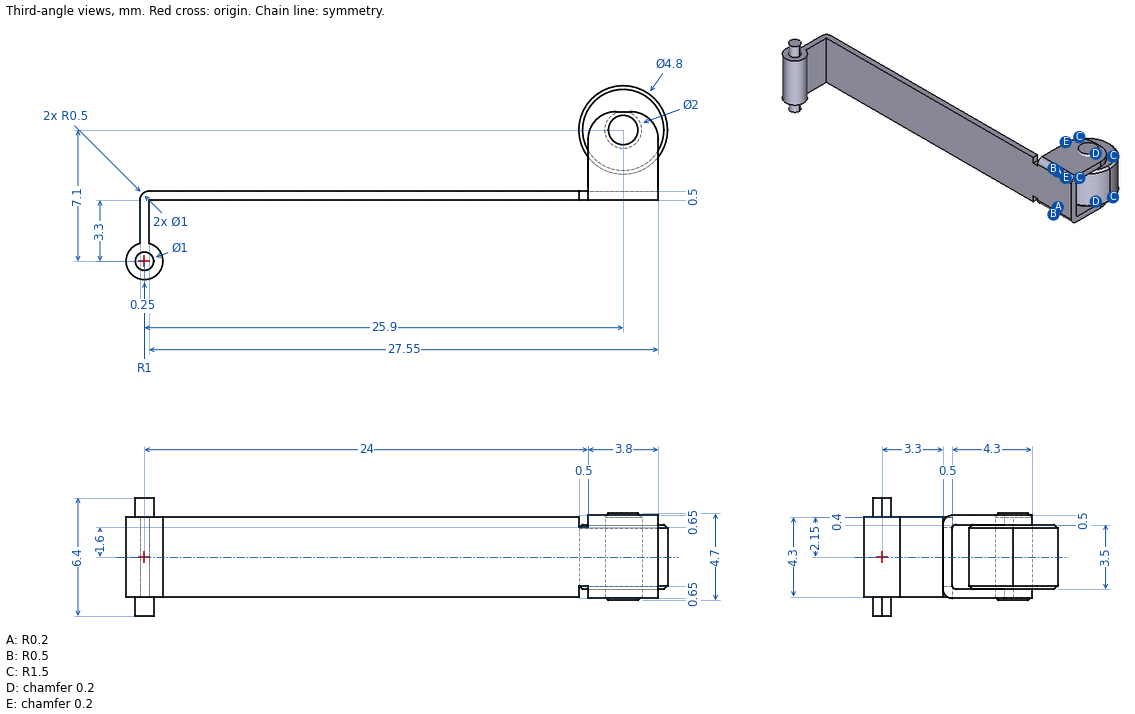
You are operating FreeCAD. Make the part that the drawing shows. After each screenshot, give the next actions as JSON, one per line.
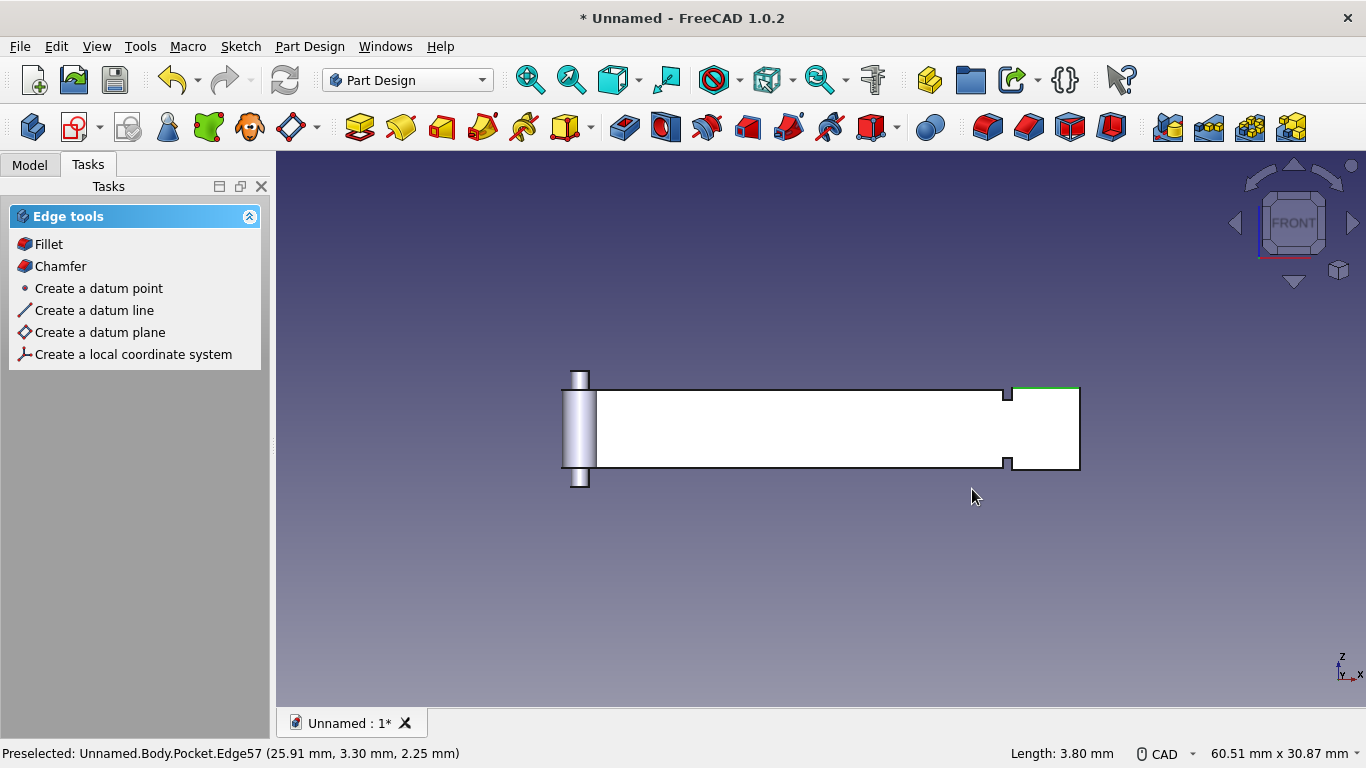
{"action": "left_click", "coordinate": [1046, 469], "text": "ctrl"}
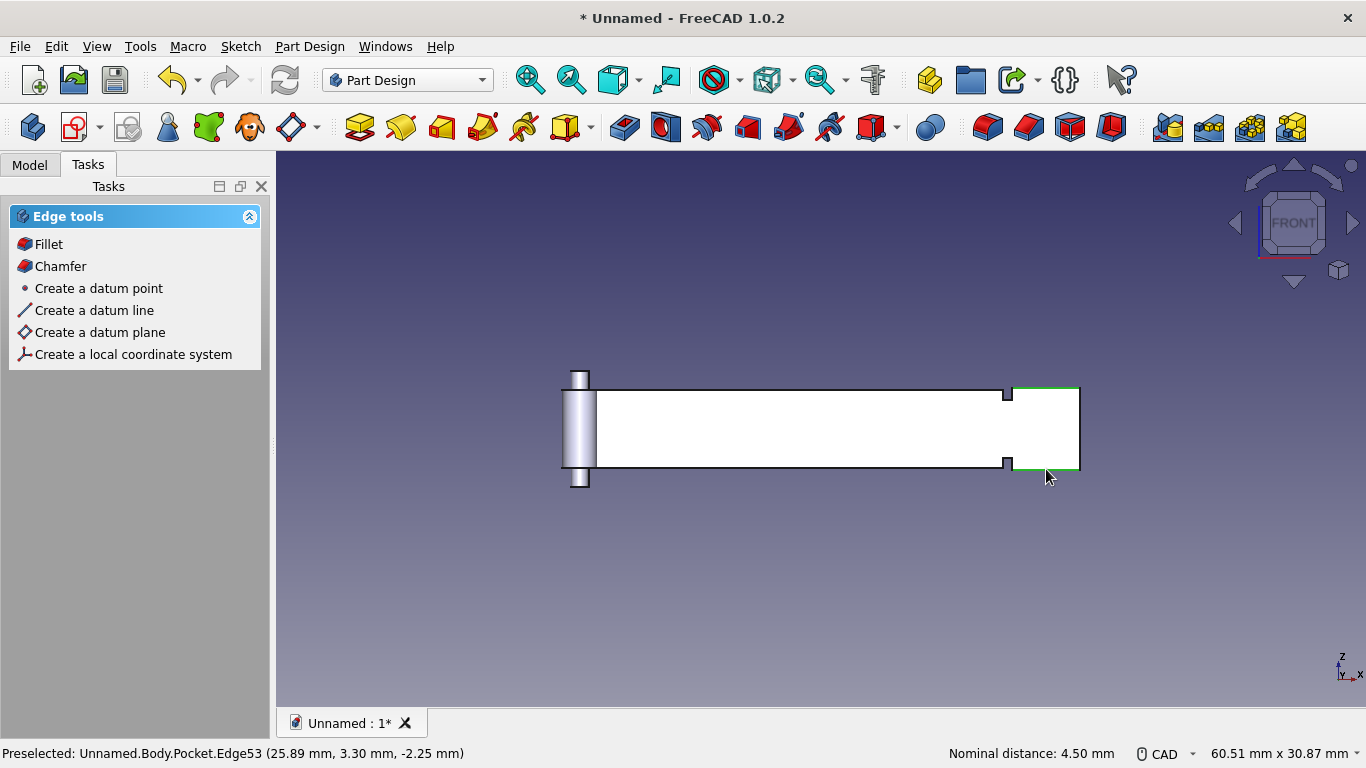
{"action": "left_click", "coordinate": [988, 128]}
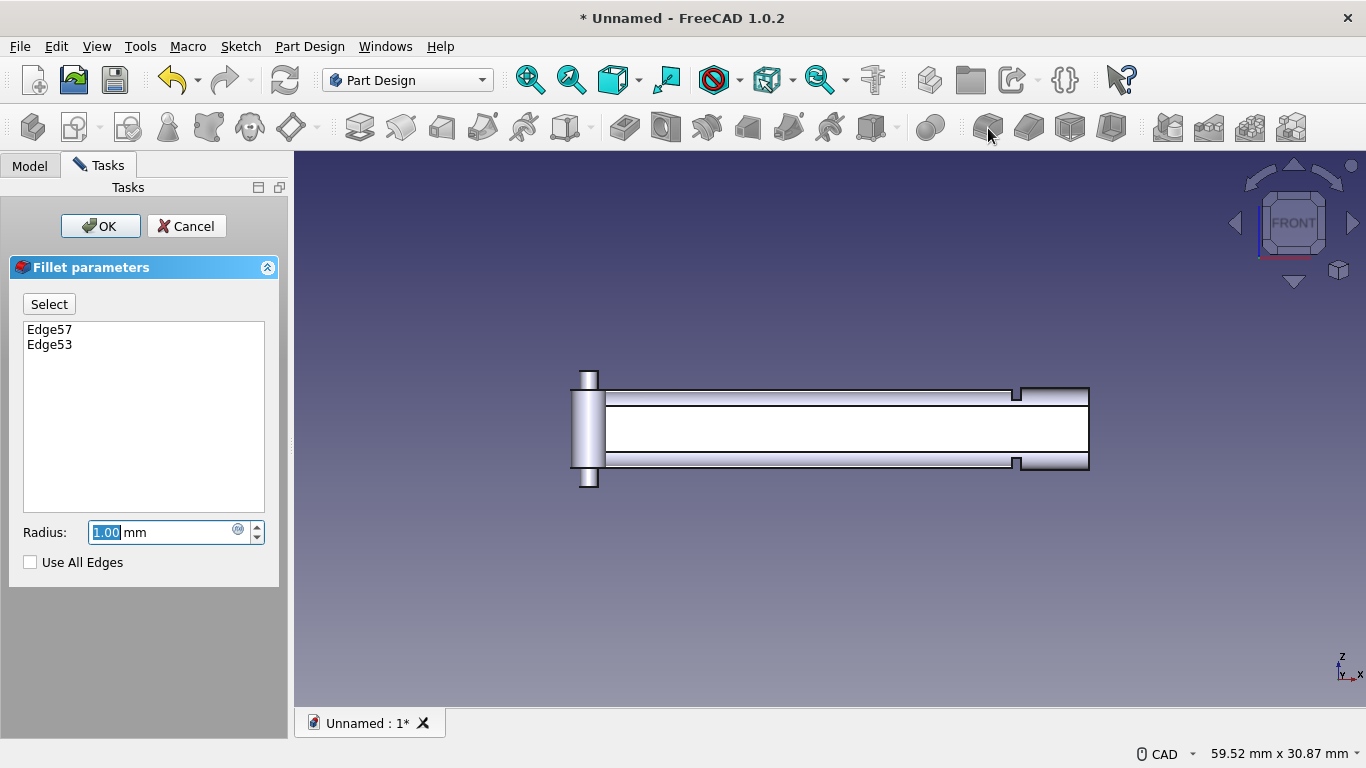
{"action": "type", "text": "0.5"}
{"action": "key", "text": "Tab"}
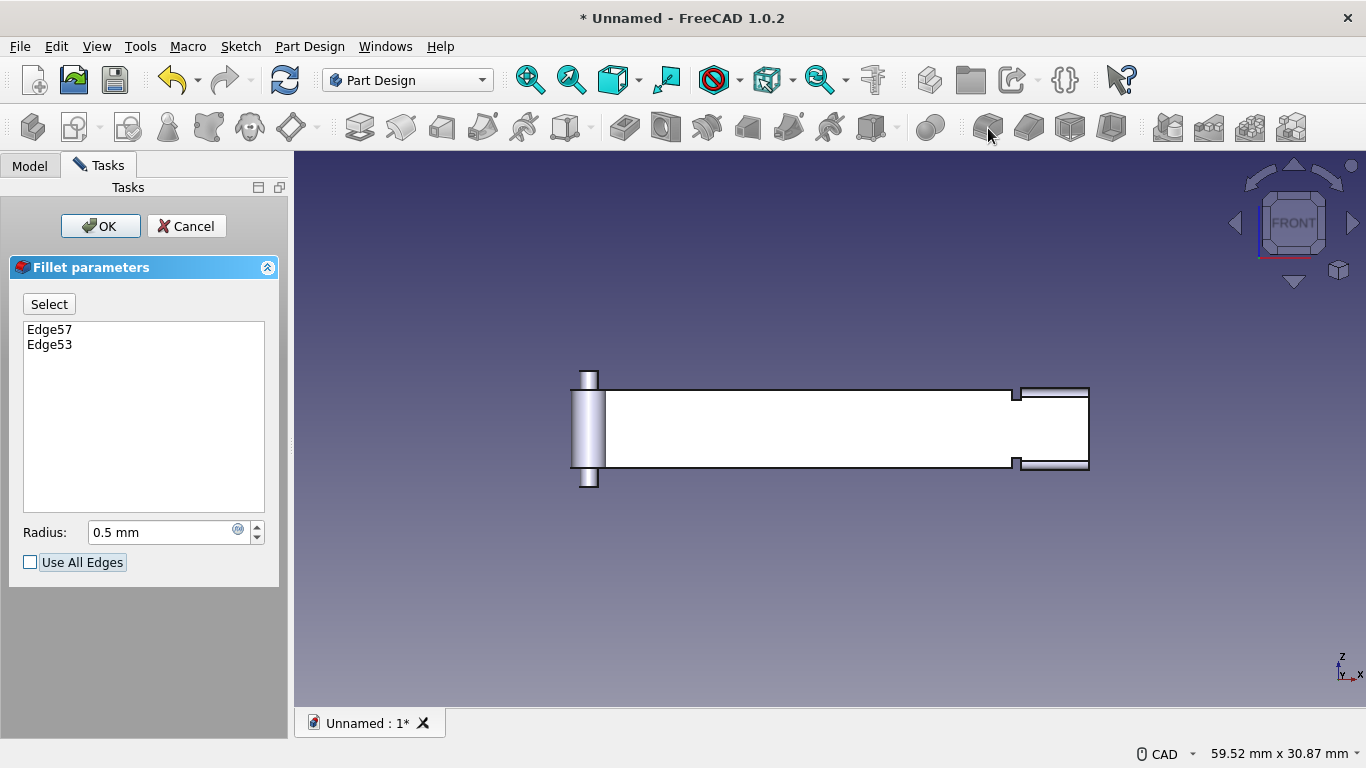
{"action": "left_click", "coordinate": [101, 226]}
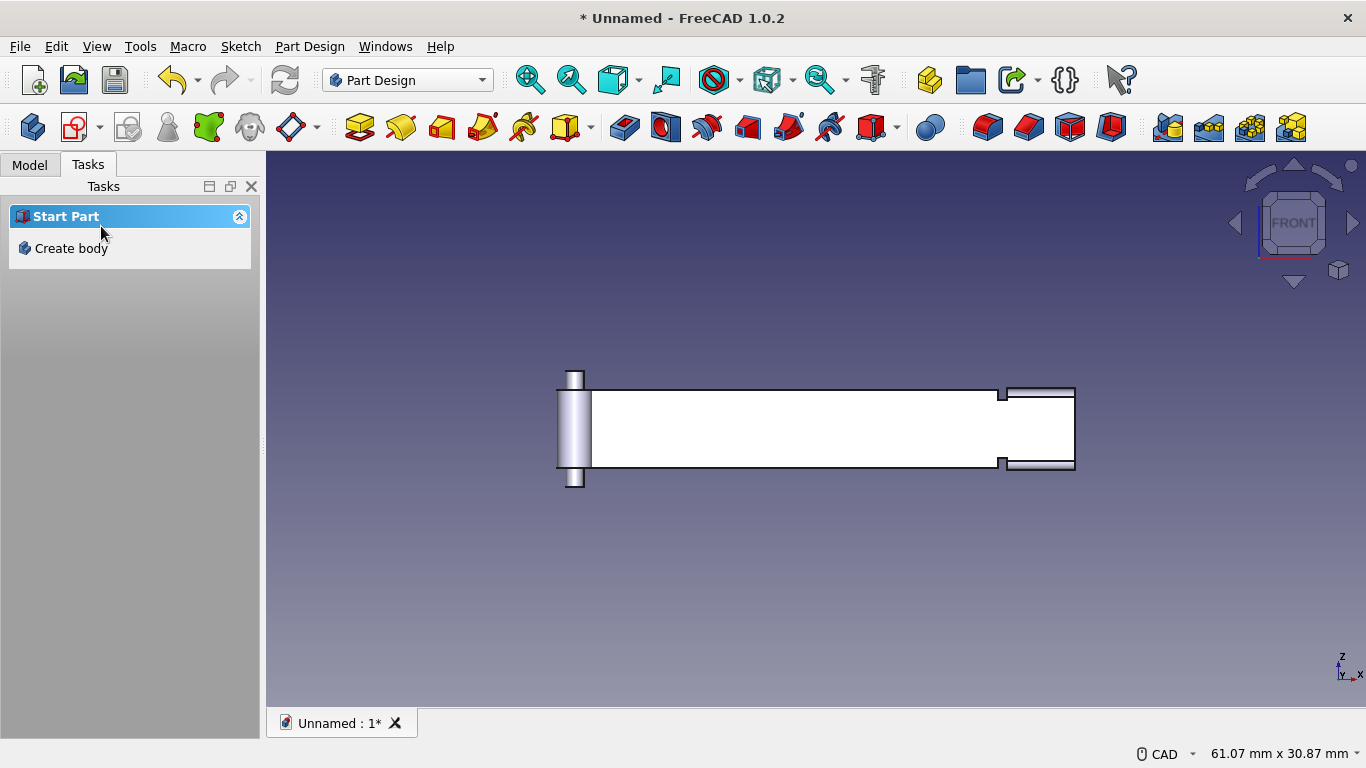
{"action": "scroll", "coordinate": [1007, 464], "scroll_direction": "up", "scroll_amount": 8}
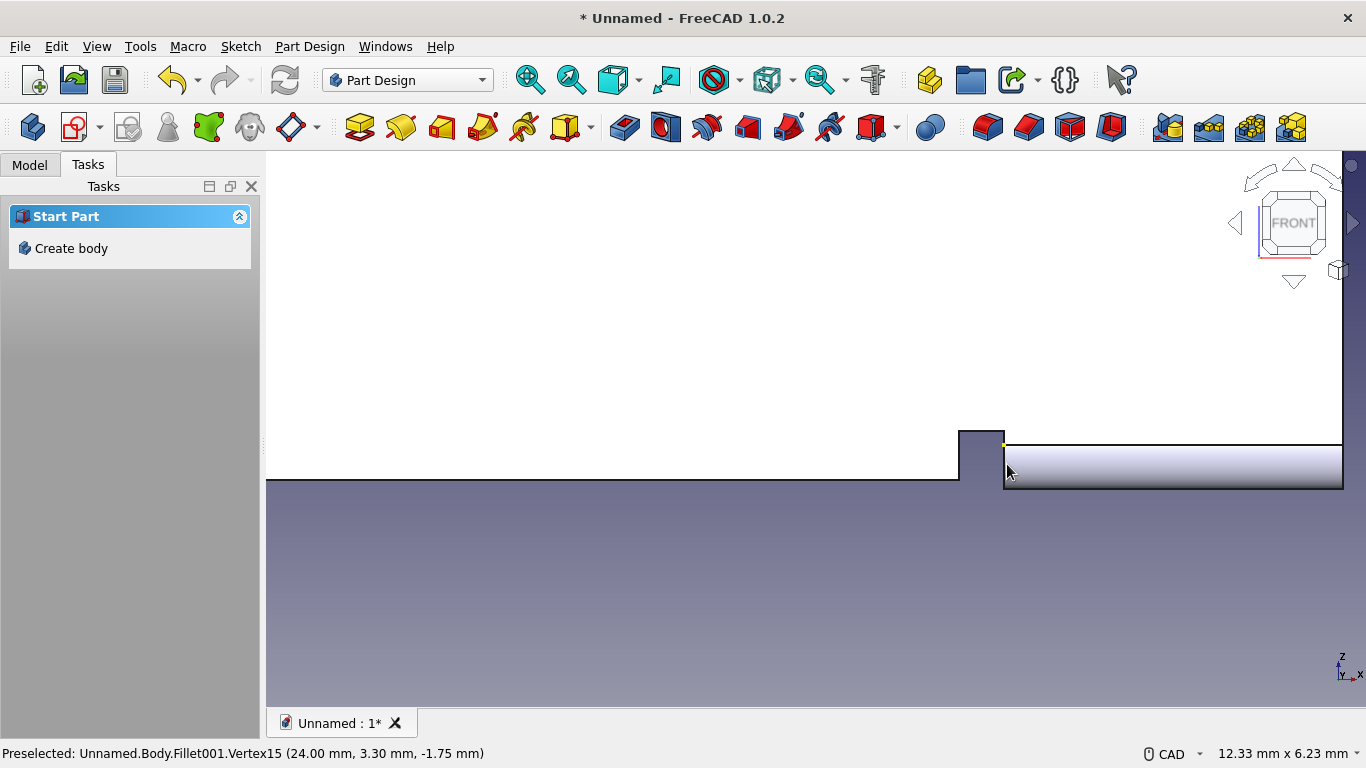
{"action": "key", "text": "v f"}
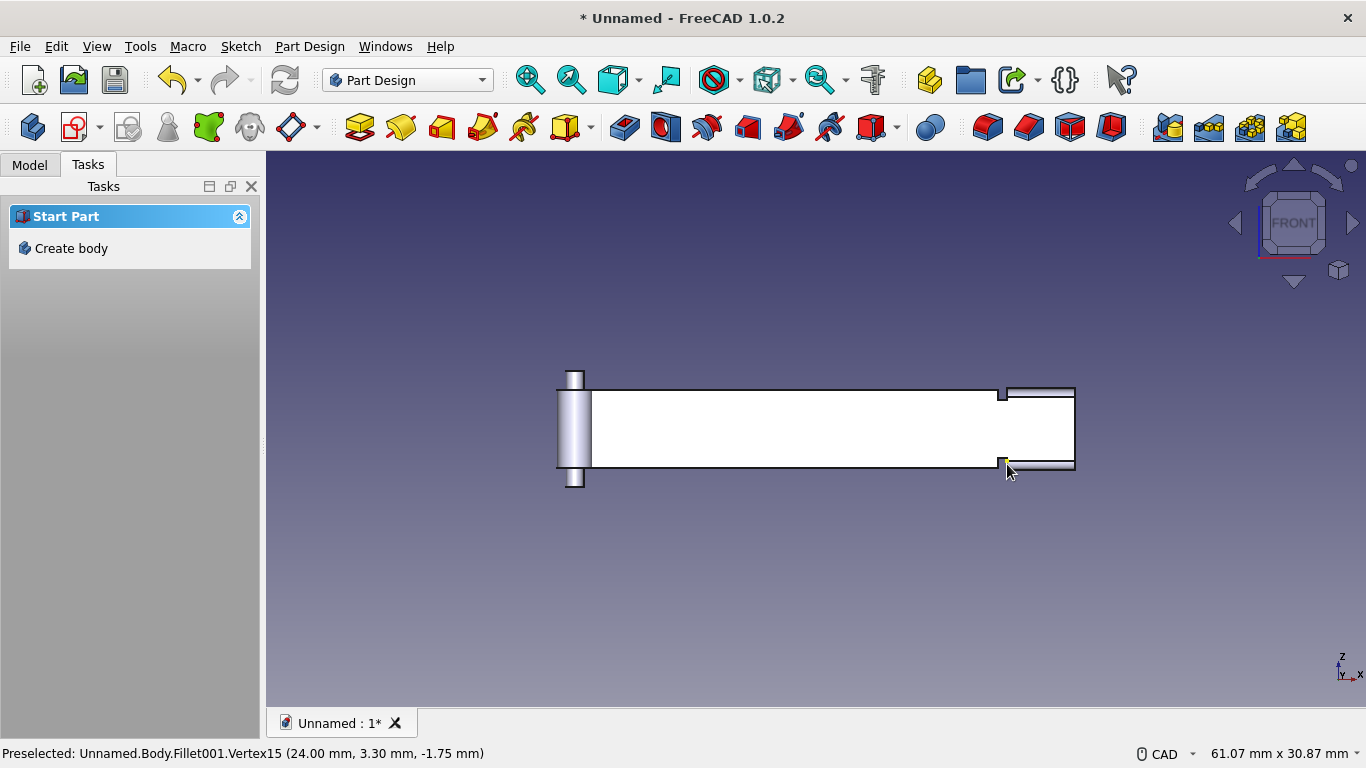
{"action": "key", "text": "0"}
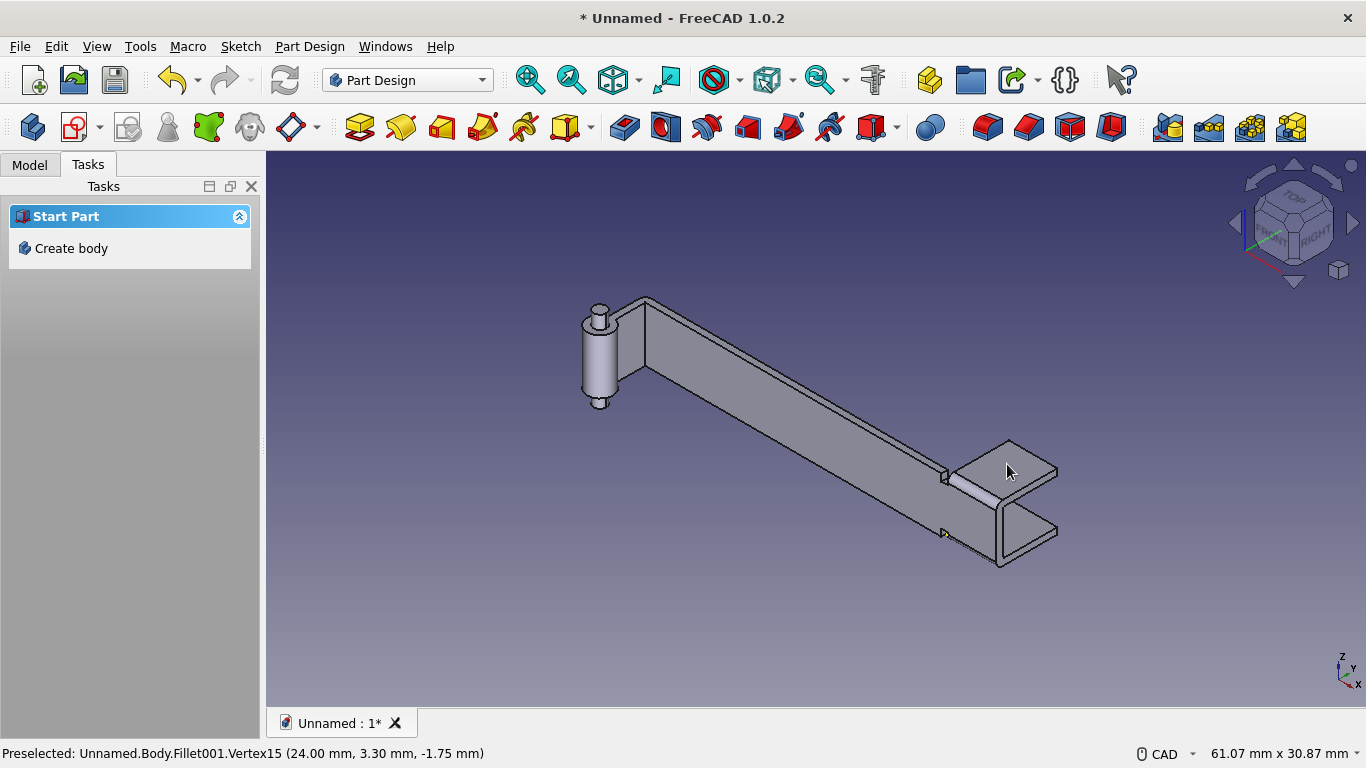
{"action": "scroll", "coordinate": [1009, 502], "scroll_direction": "up", "scroll_amount": 8}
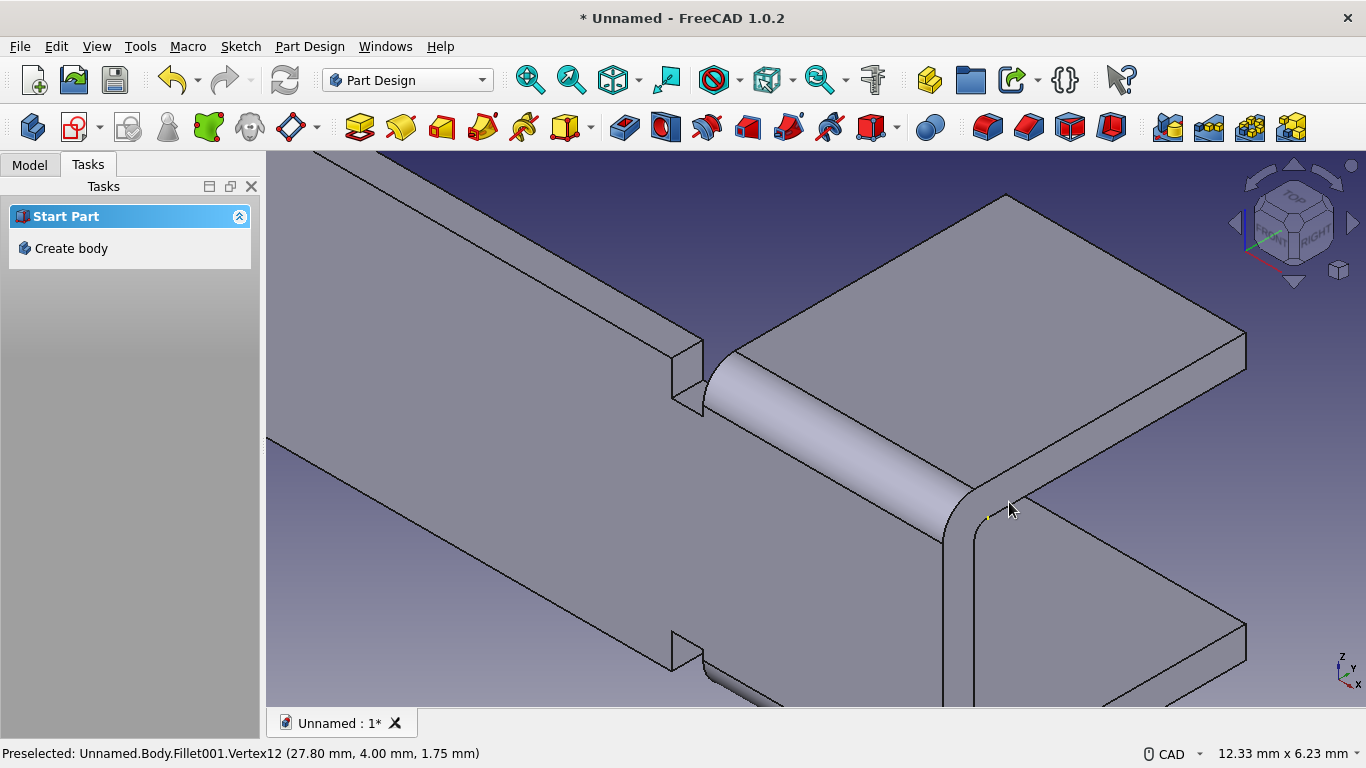
{"action": "left_click", "coordinate": [531, 80]}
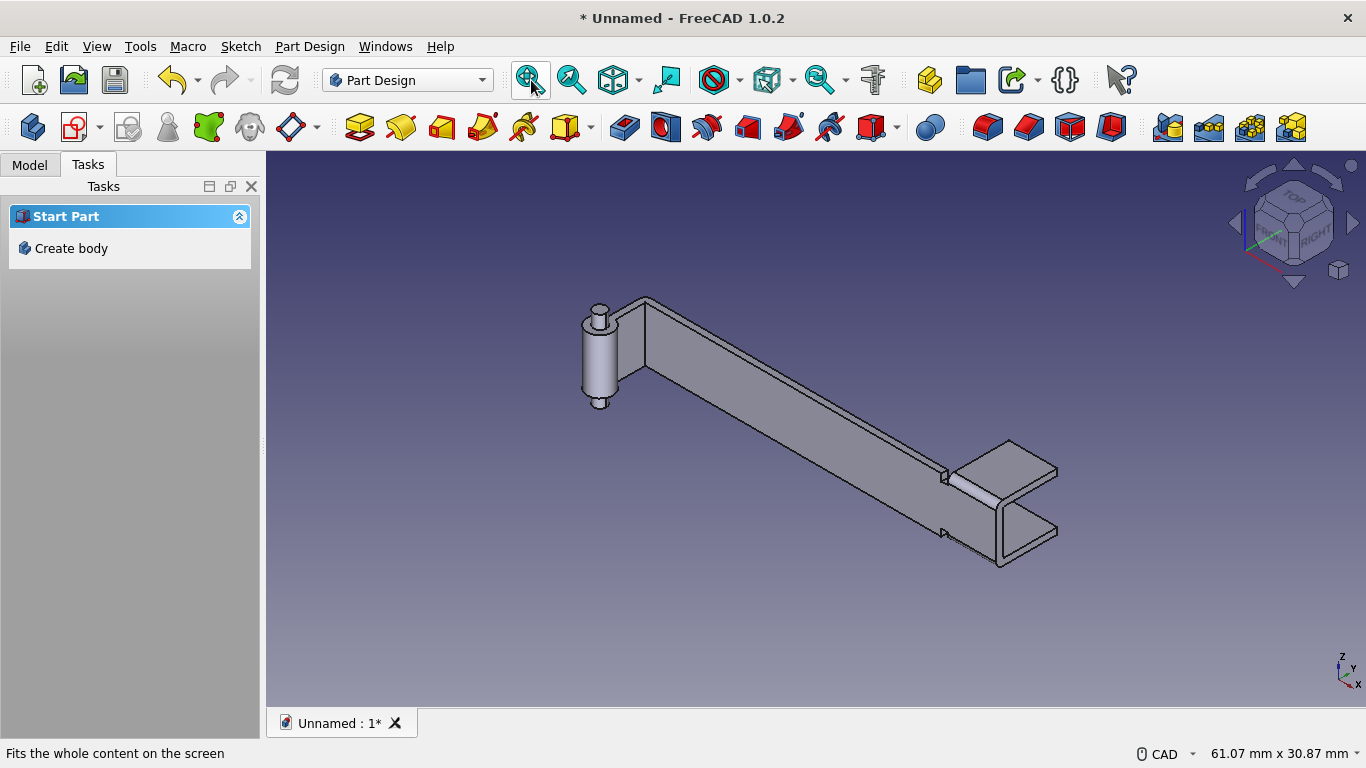
{"action": "key", "text": "2"}